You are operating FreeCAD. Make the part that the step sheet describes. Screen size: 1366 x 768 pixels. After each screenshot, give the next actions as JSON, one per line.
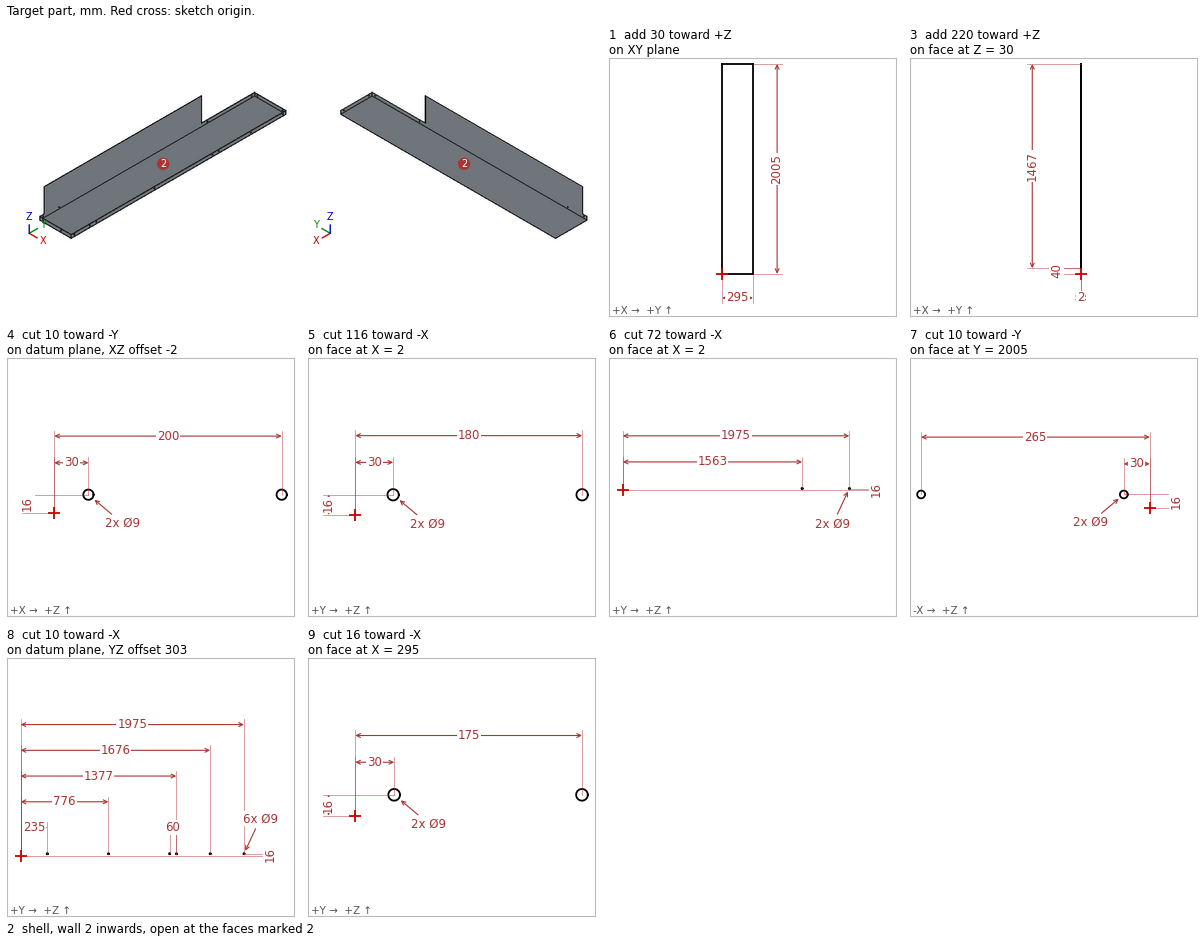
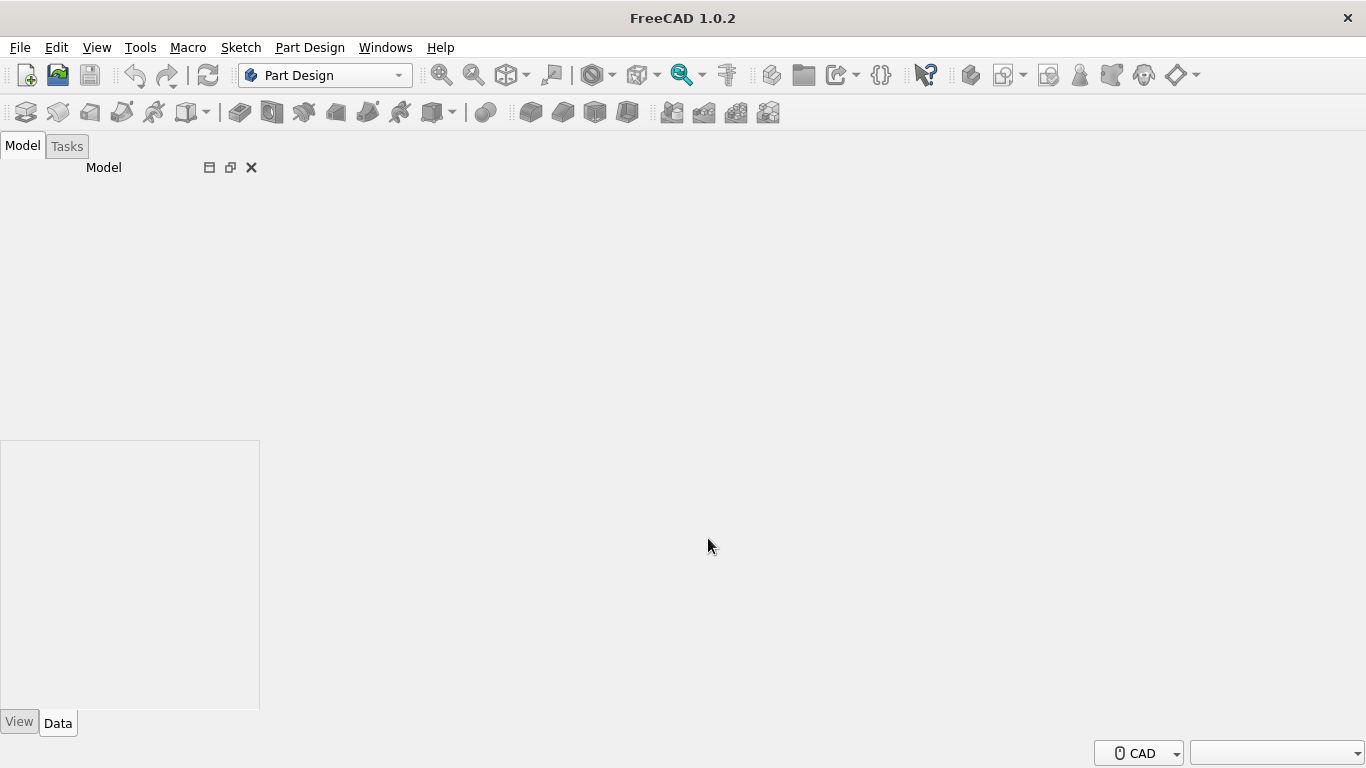
{"action": "left_click", "coordinate": [26, 76]}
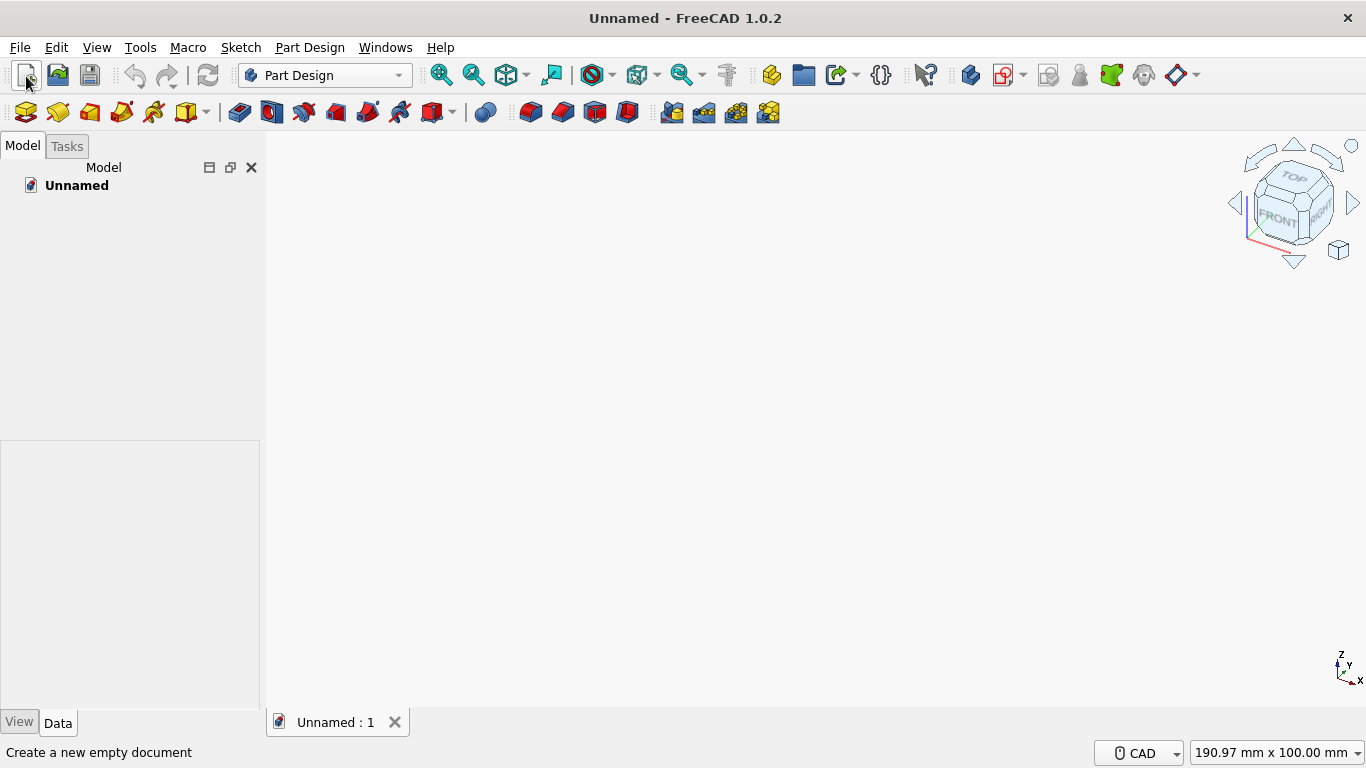
{"action": "left_click", "coordinate": [1004, 76]}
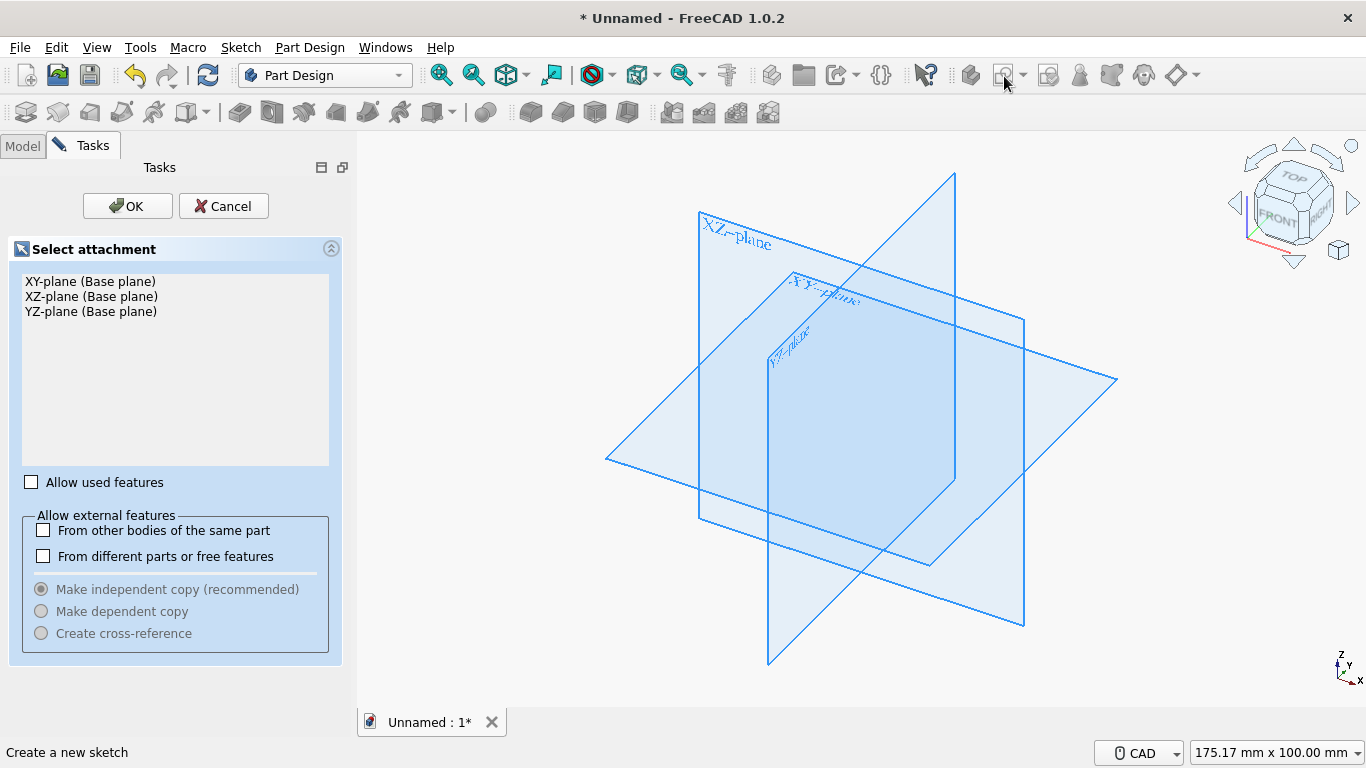
{"action": "left_click", "coordinate": [82, 282]}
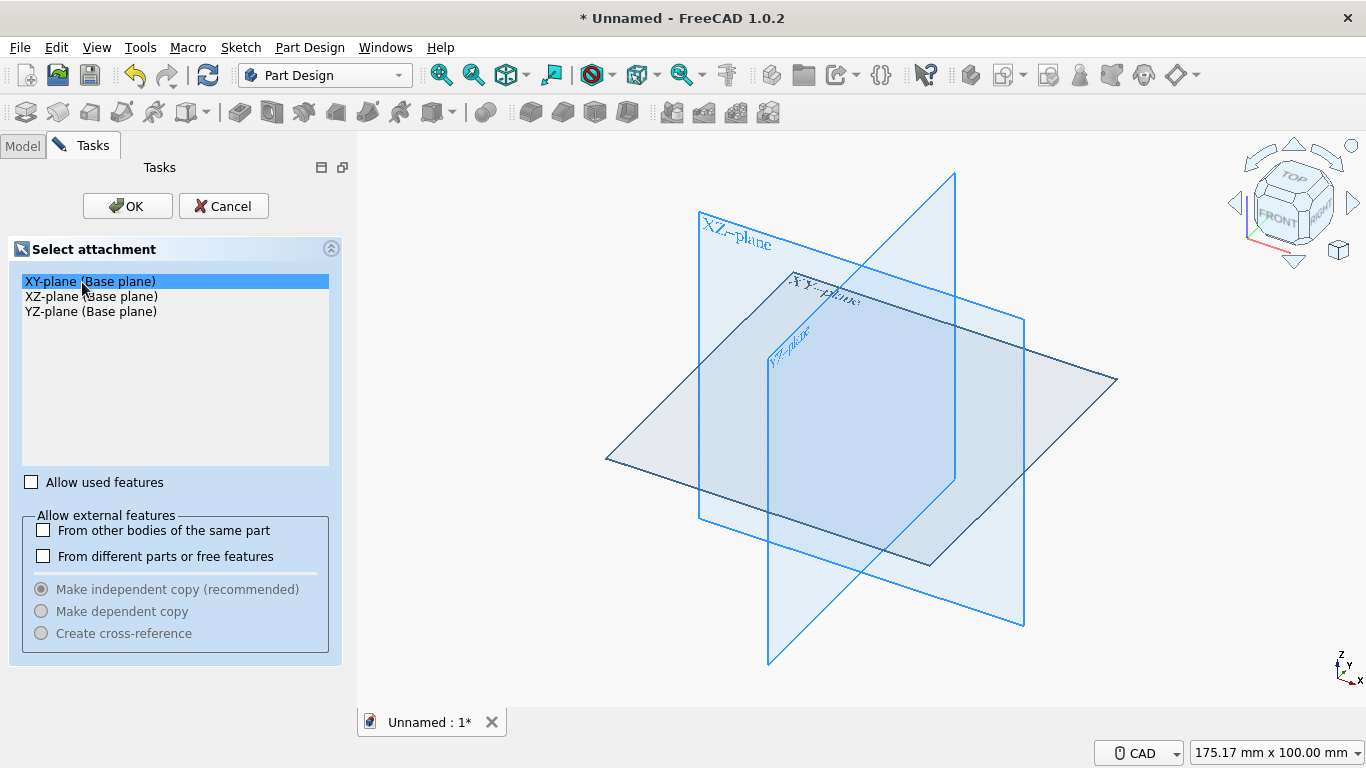
{"action": "left_click", "coordinate": [128, 206]}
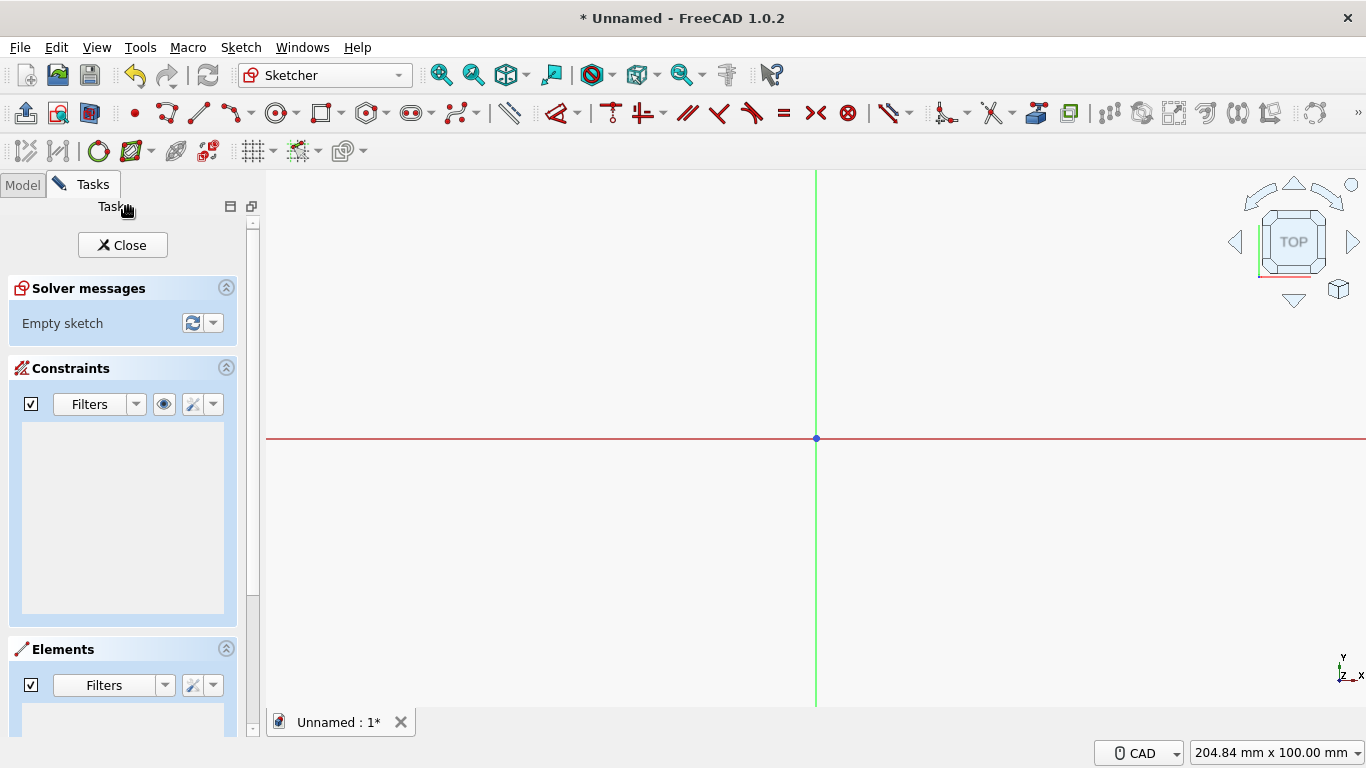
{"action": "scroll", "coordinate": [718, 624], "scroll_direction": "down", "scroll_amount": 17}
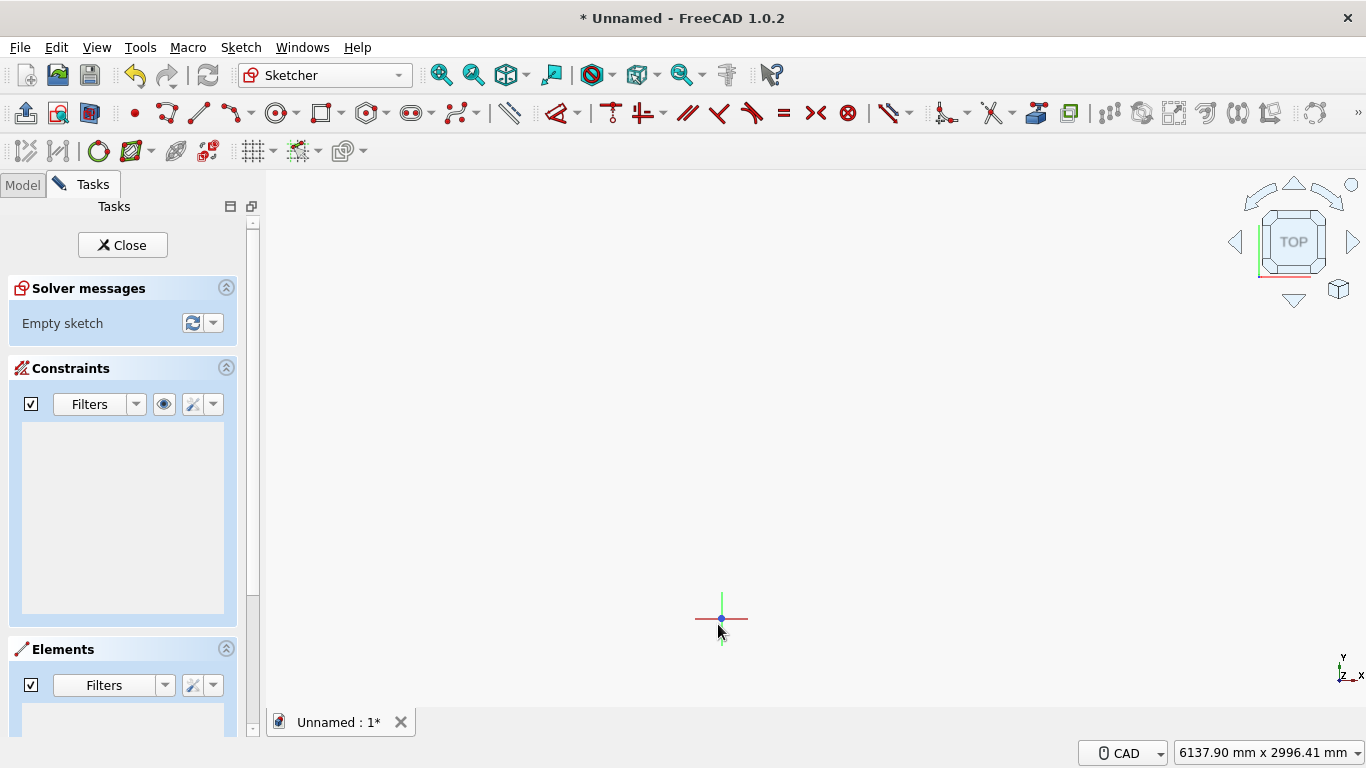
{"action": "left_click", "coordinate": [322, 114]}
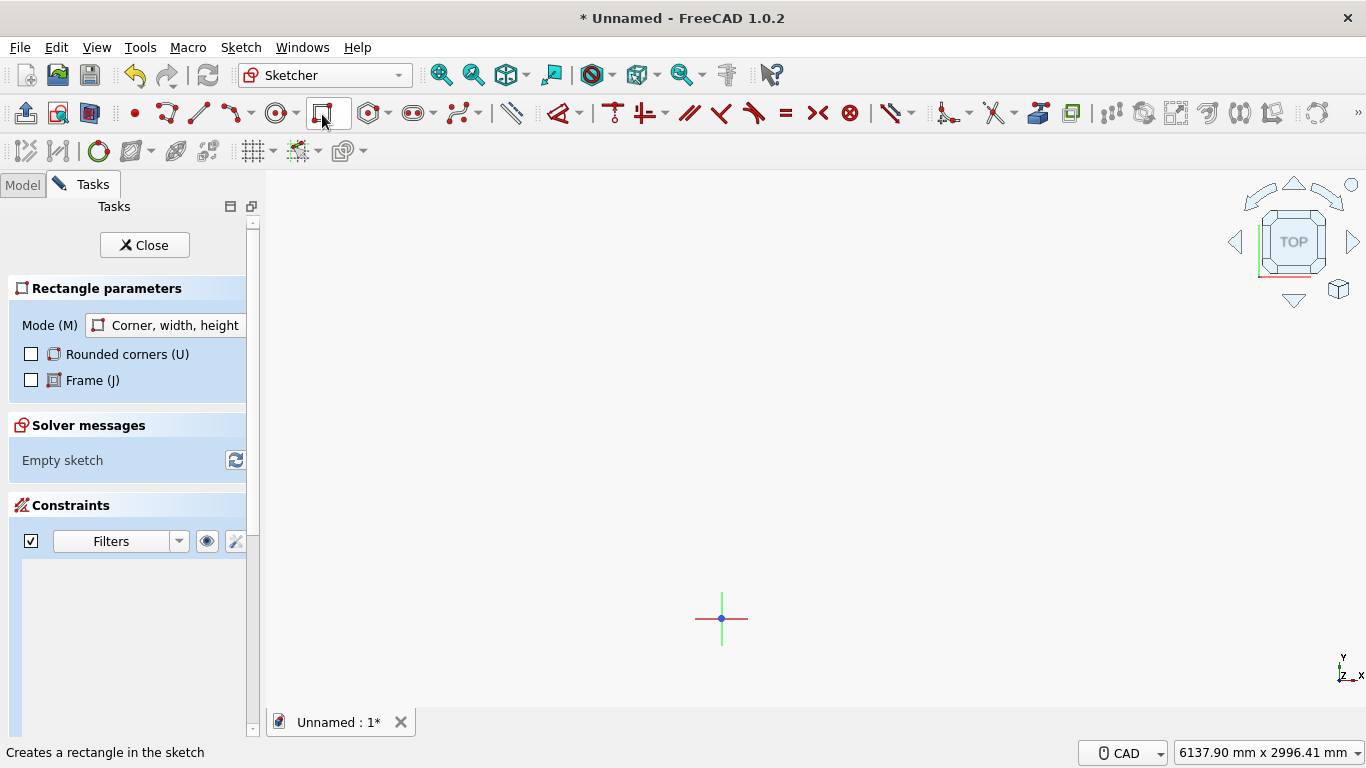
{"action": "left_click", "coordinate": [722, 619]}
{"action": "left_click", "coordinate": [775, 259]}
{"action": "key", "text": "Escape"}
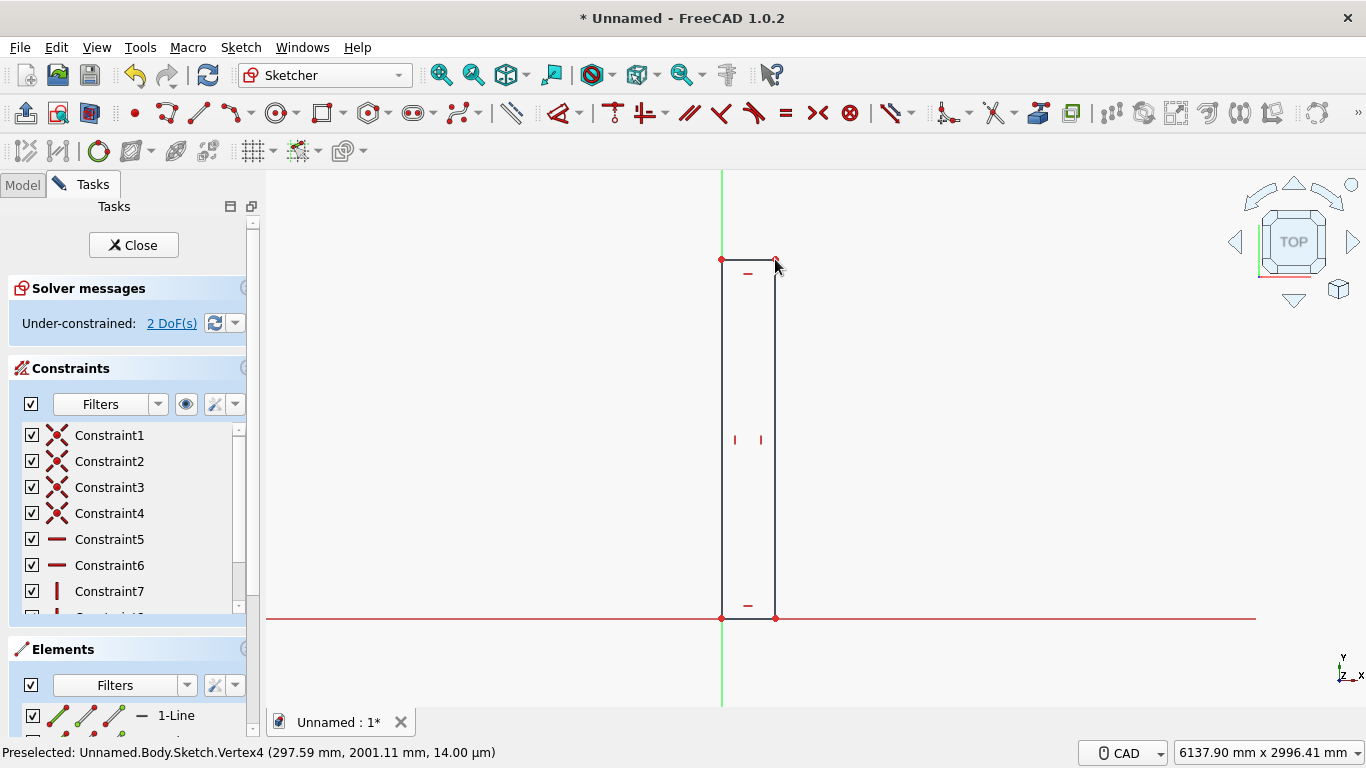
{"action": "left_click", "coordinate": [558, 114]}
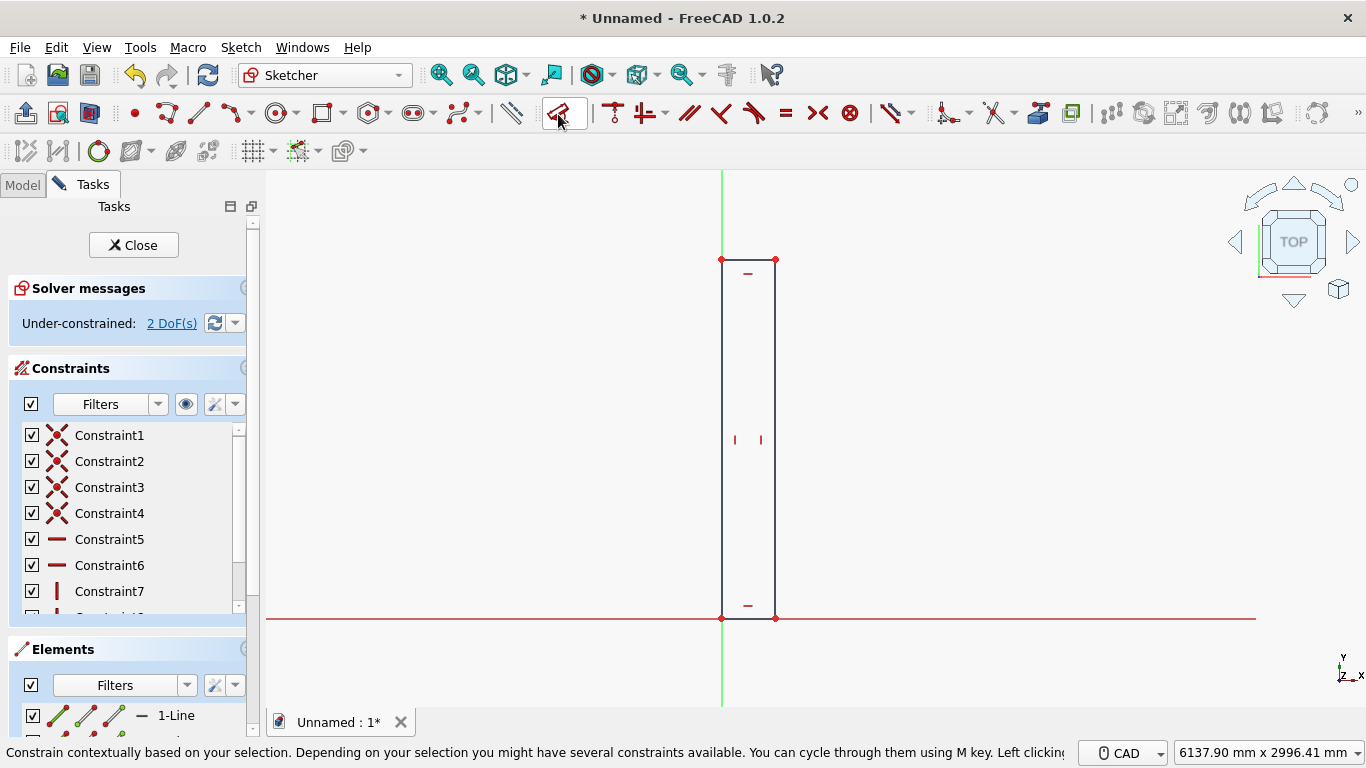
{"action": "left_click", "coordinate": [738, 619]}
{"action": "left_click", "coordinate": [748, 653]}